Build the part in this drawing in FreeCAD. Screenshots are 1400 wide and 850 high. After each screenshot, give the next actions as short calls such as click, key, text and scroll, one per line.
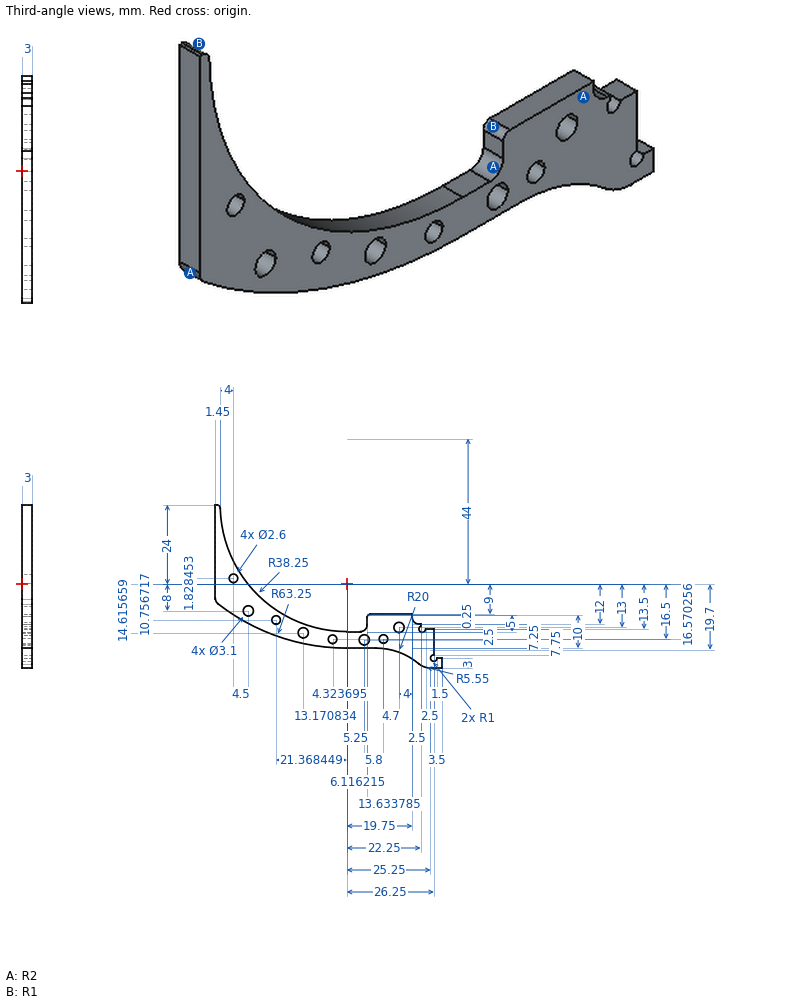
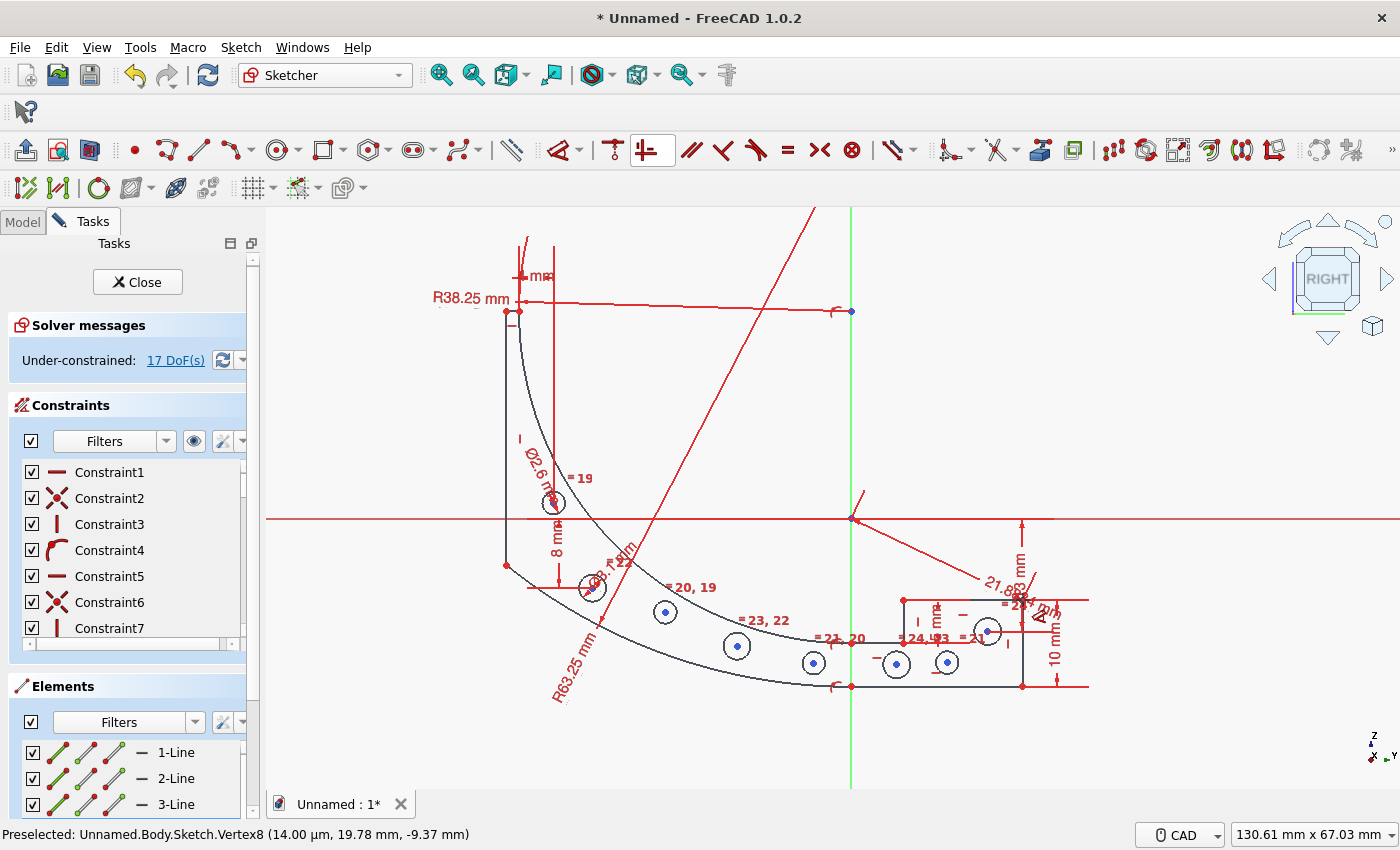
click(988, 632)
click(1005, 666)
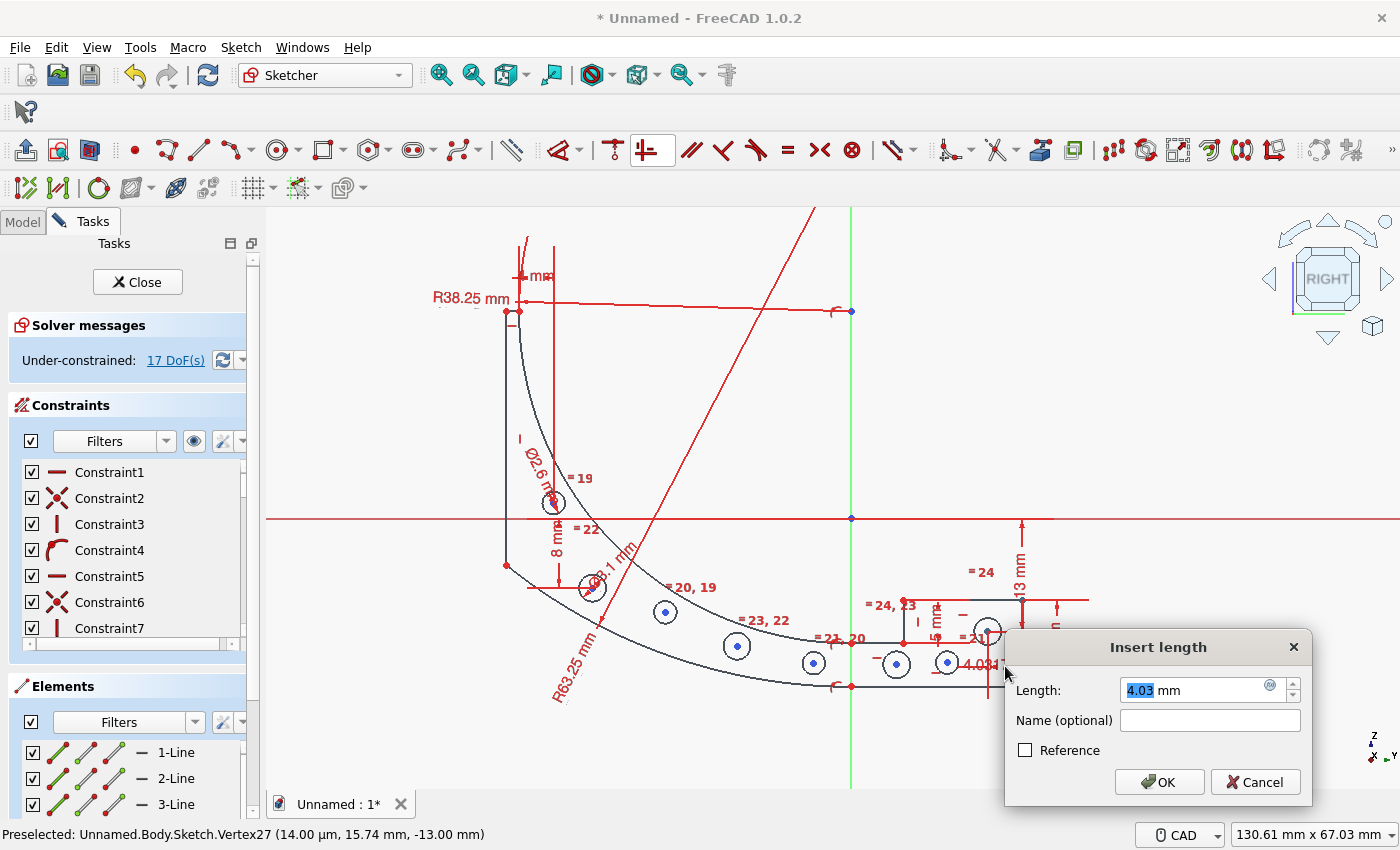
text(4)
key(Return)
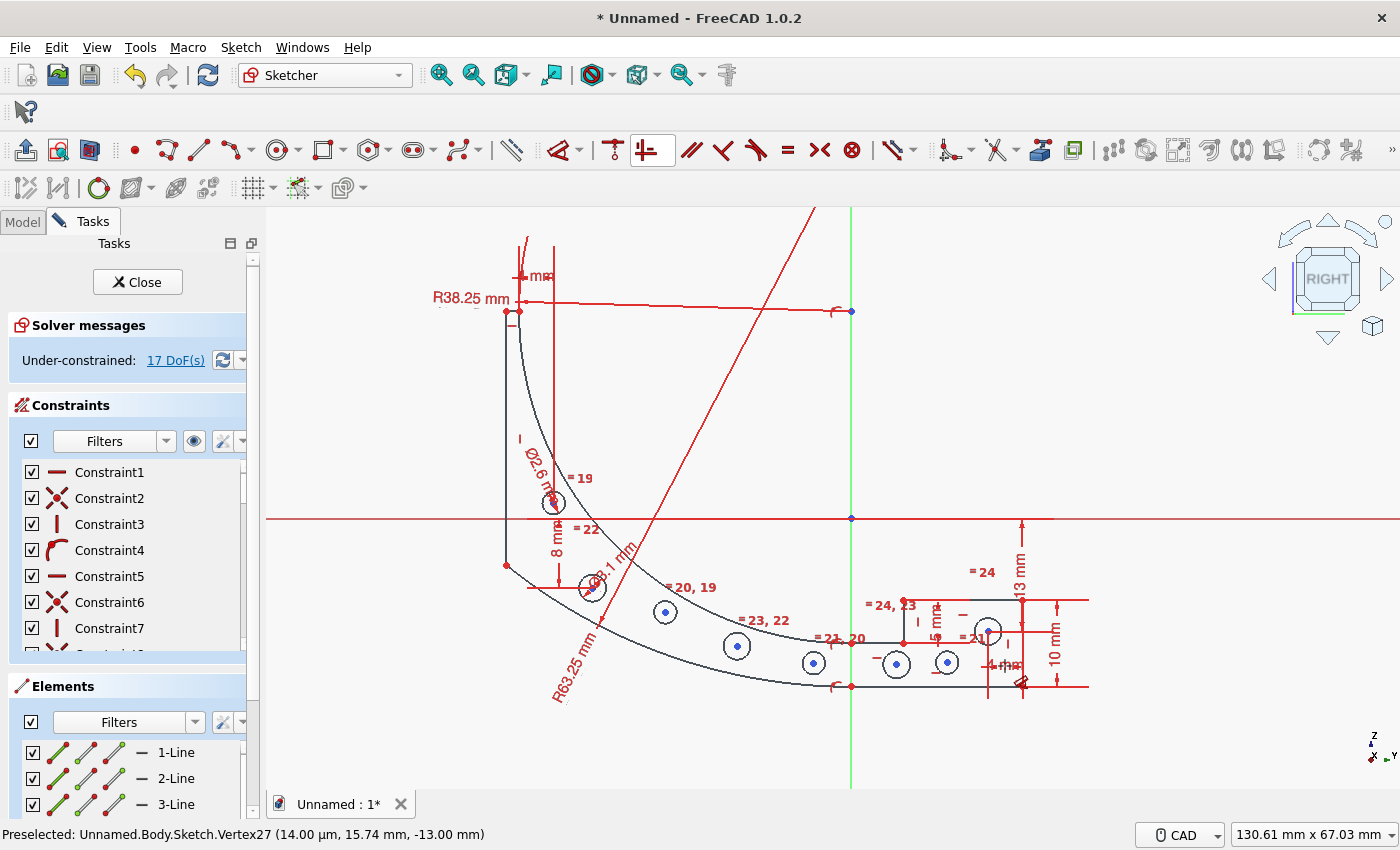
click(519, 311)
click(485, 415)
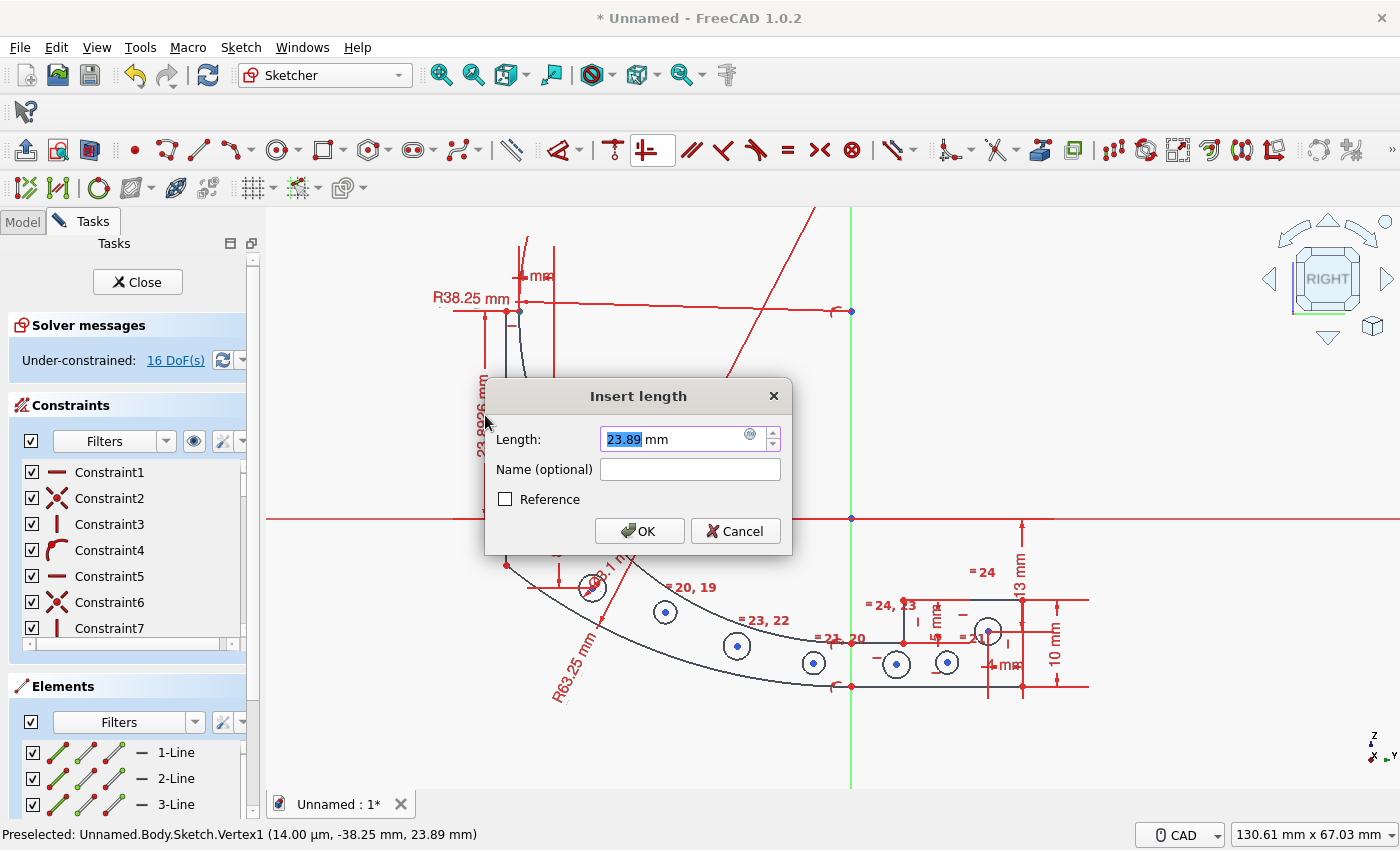
text(24)
key(Return)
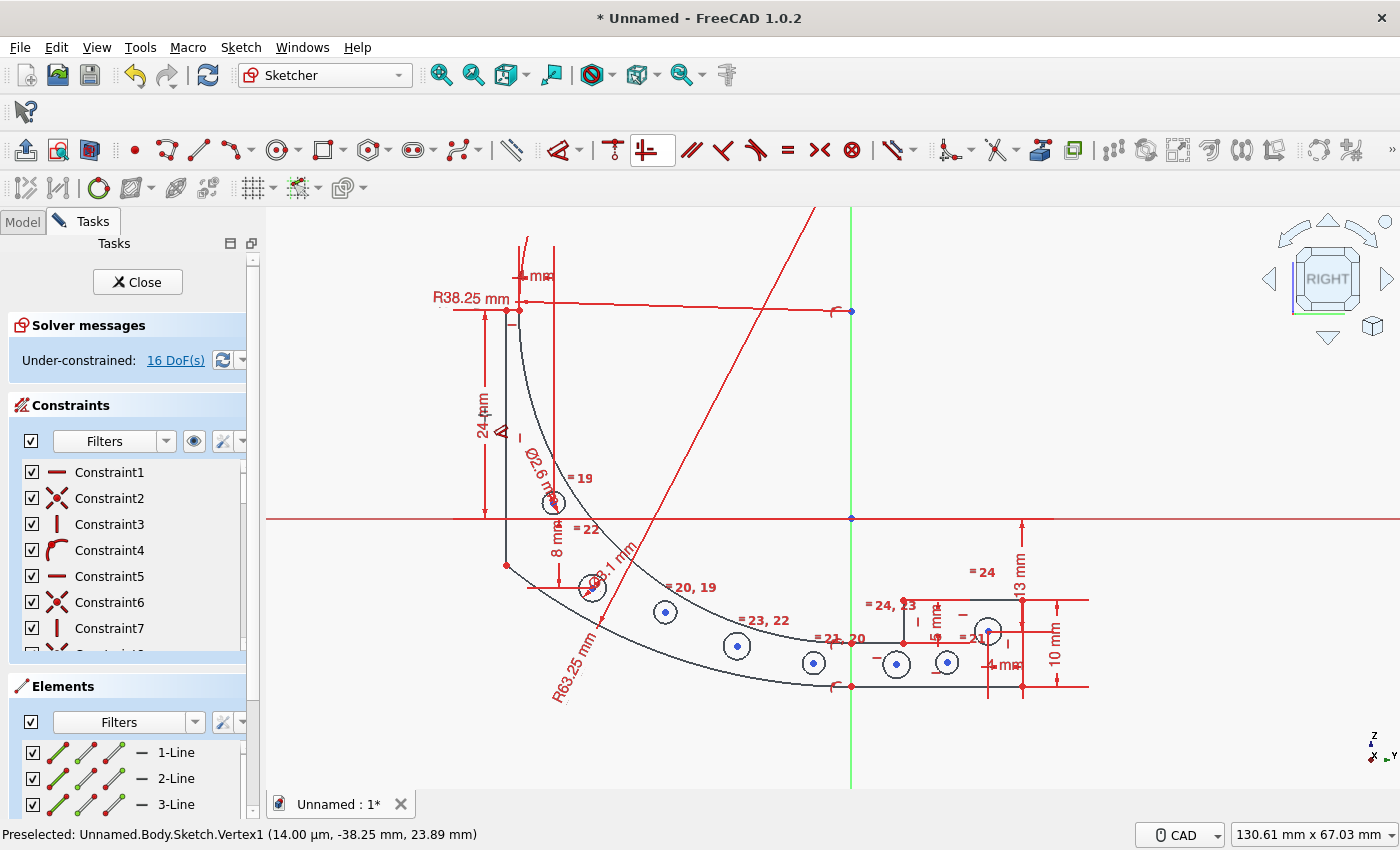
scroll(764, 673, down, 2)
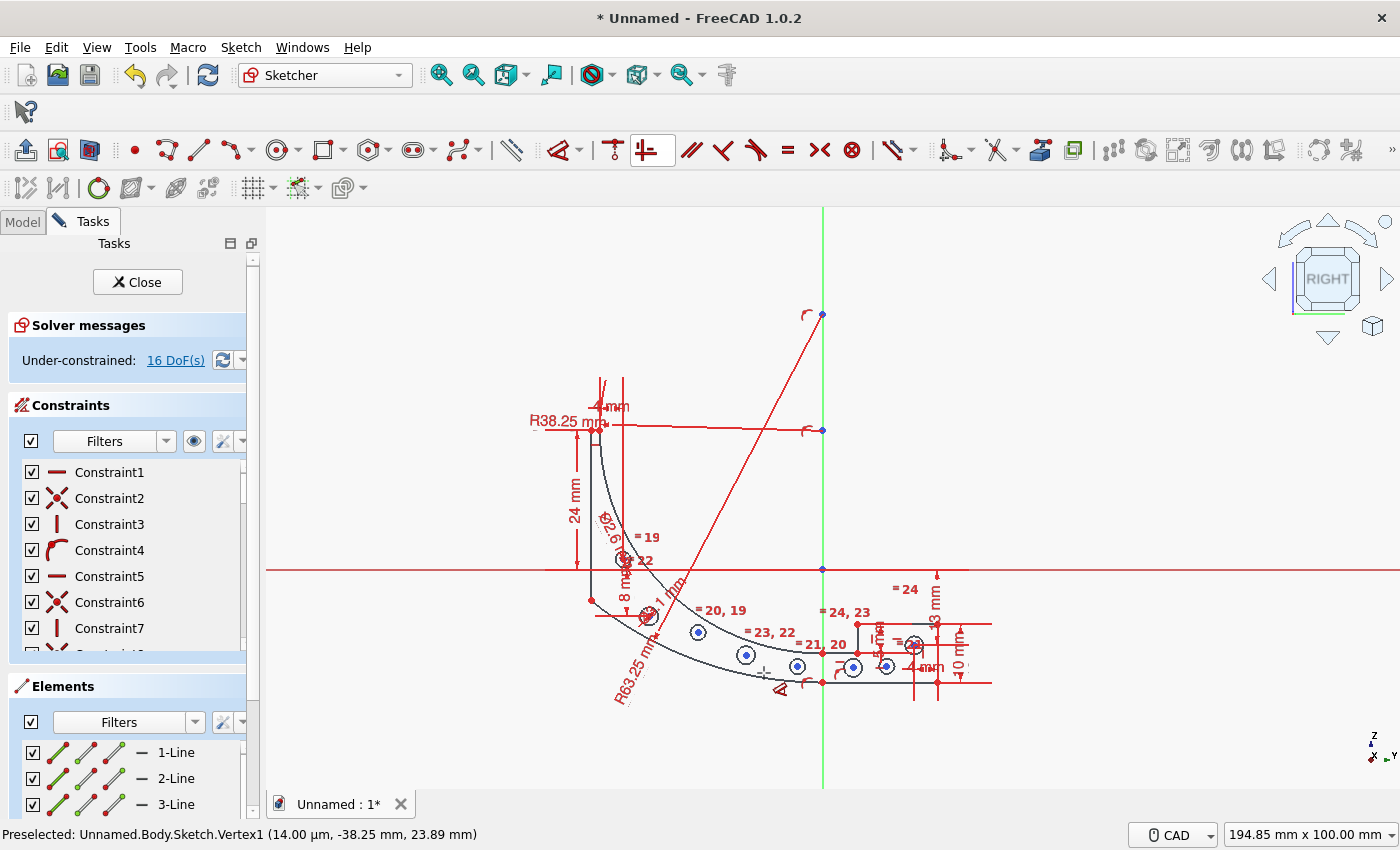
click(823, 314)
click(857, 442)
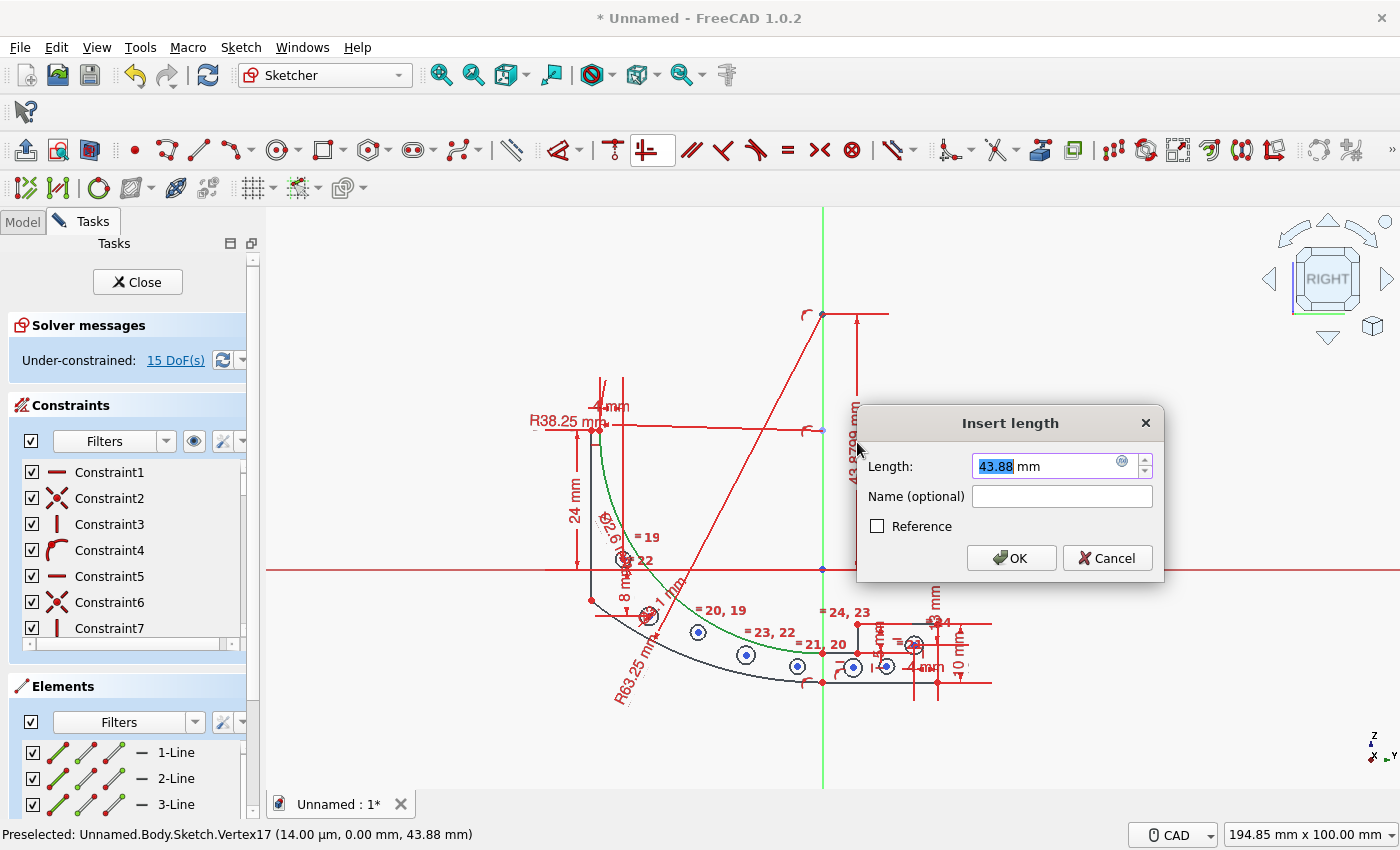
text(44)
key(Return)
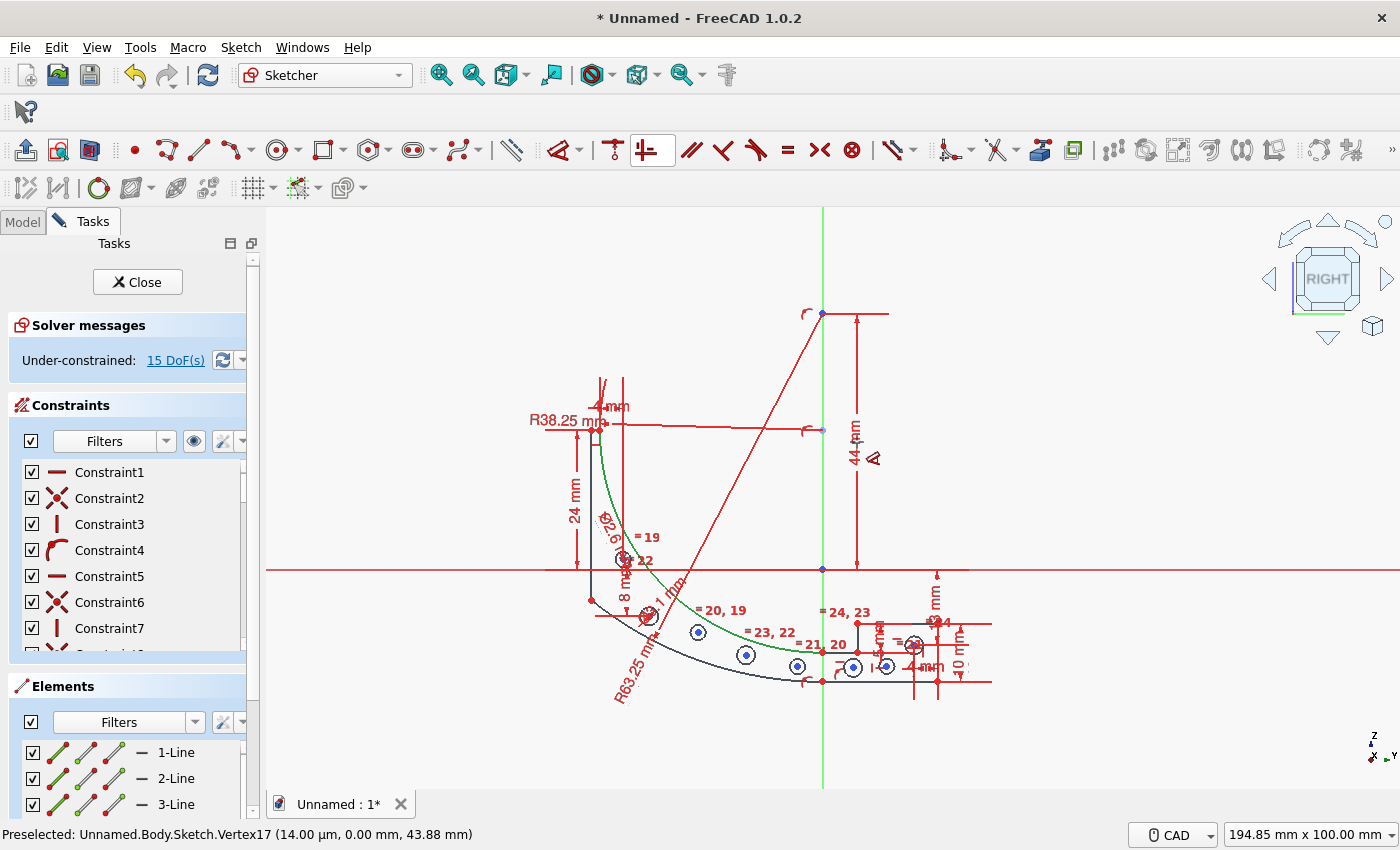
scroll(596, 430, up, 8)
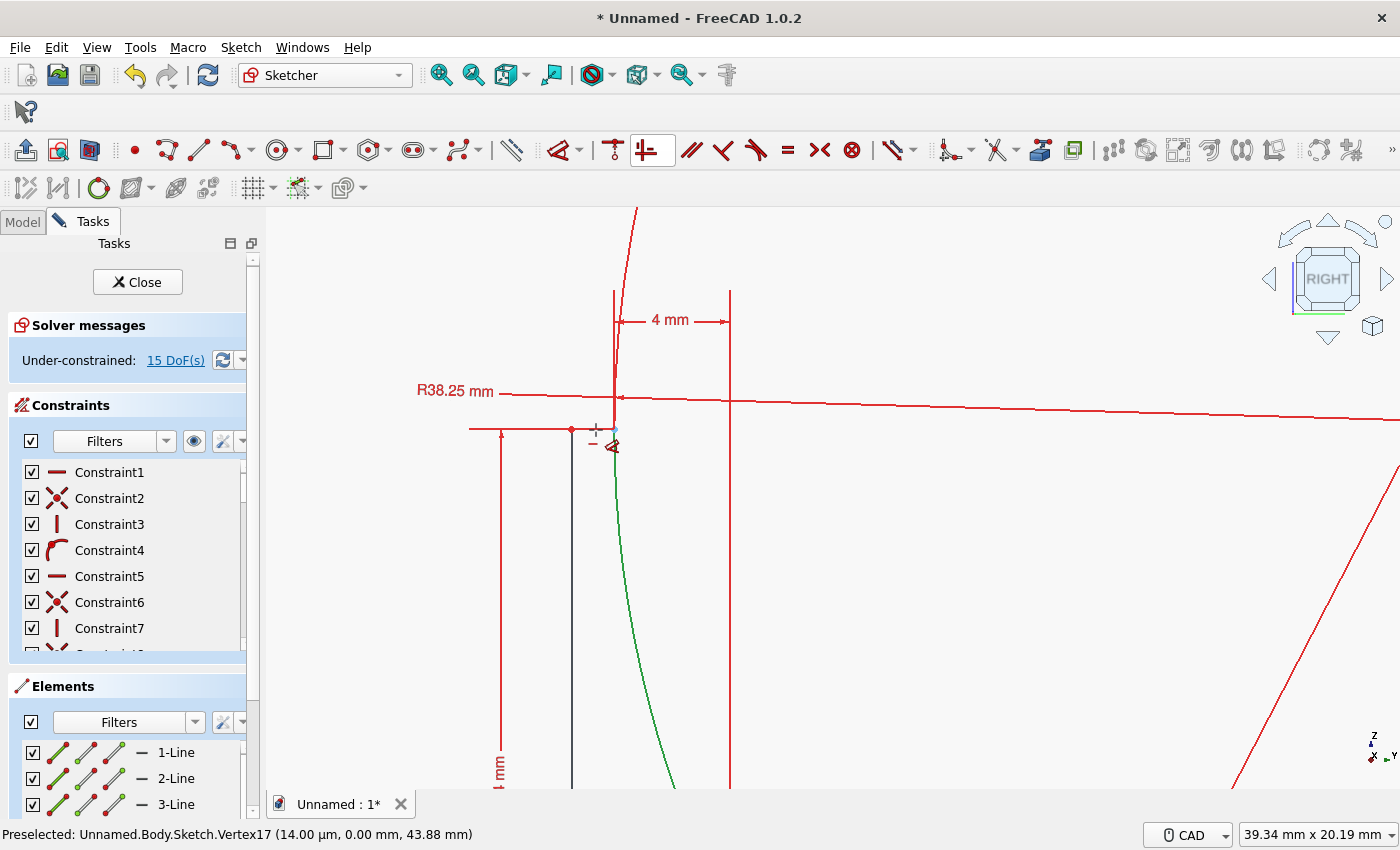
click(593, 429)
click(593, 395)